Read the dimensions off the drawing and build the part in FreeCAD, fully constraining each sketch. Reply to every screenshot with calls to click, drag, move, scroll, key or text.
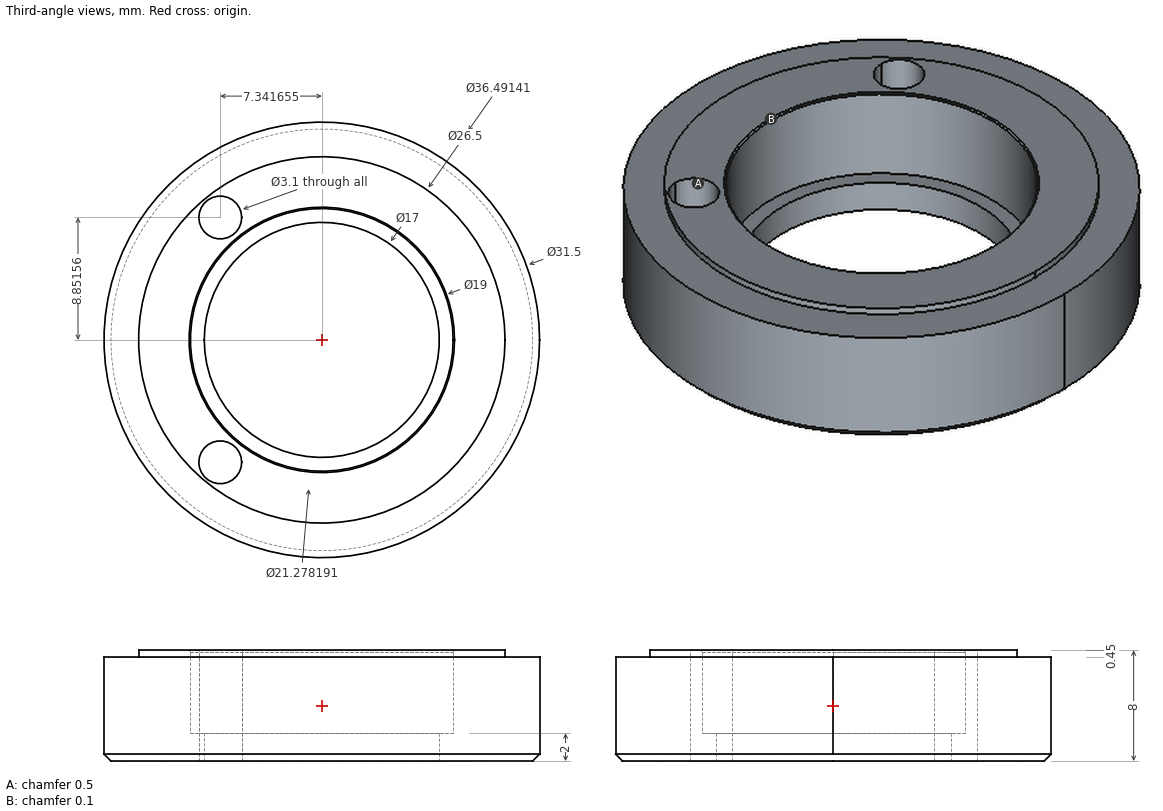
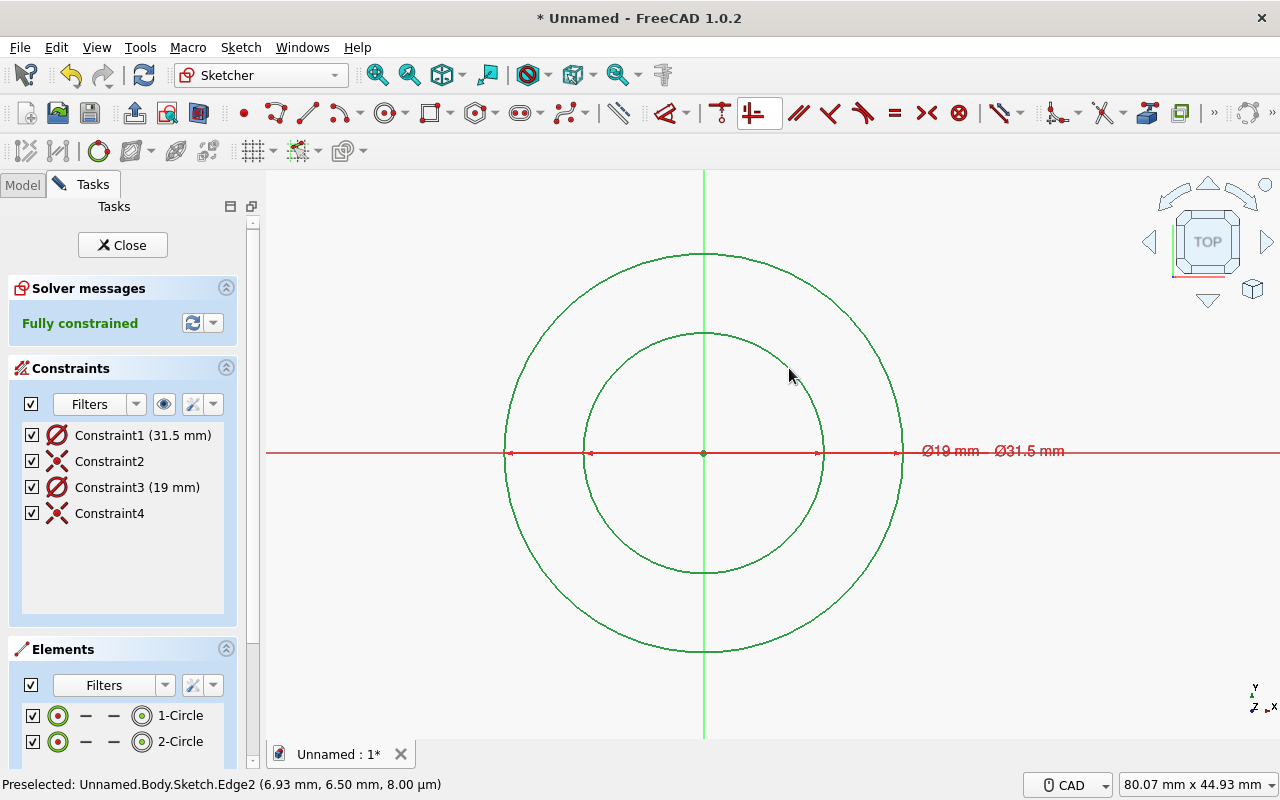
click(123, 245)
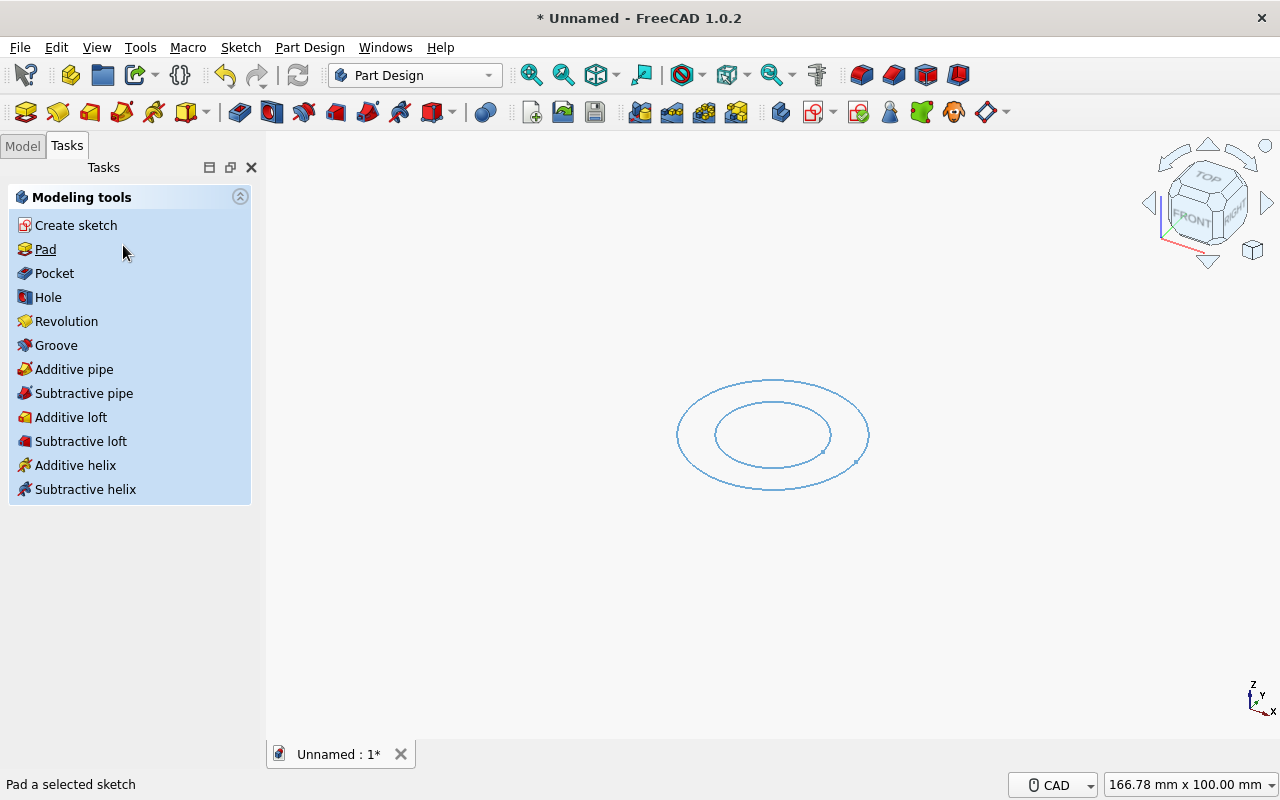
click(26, 112)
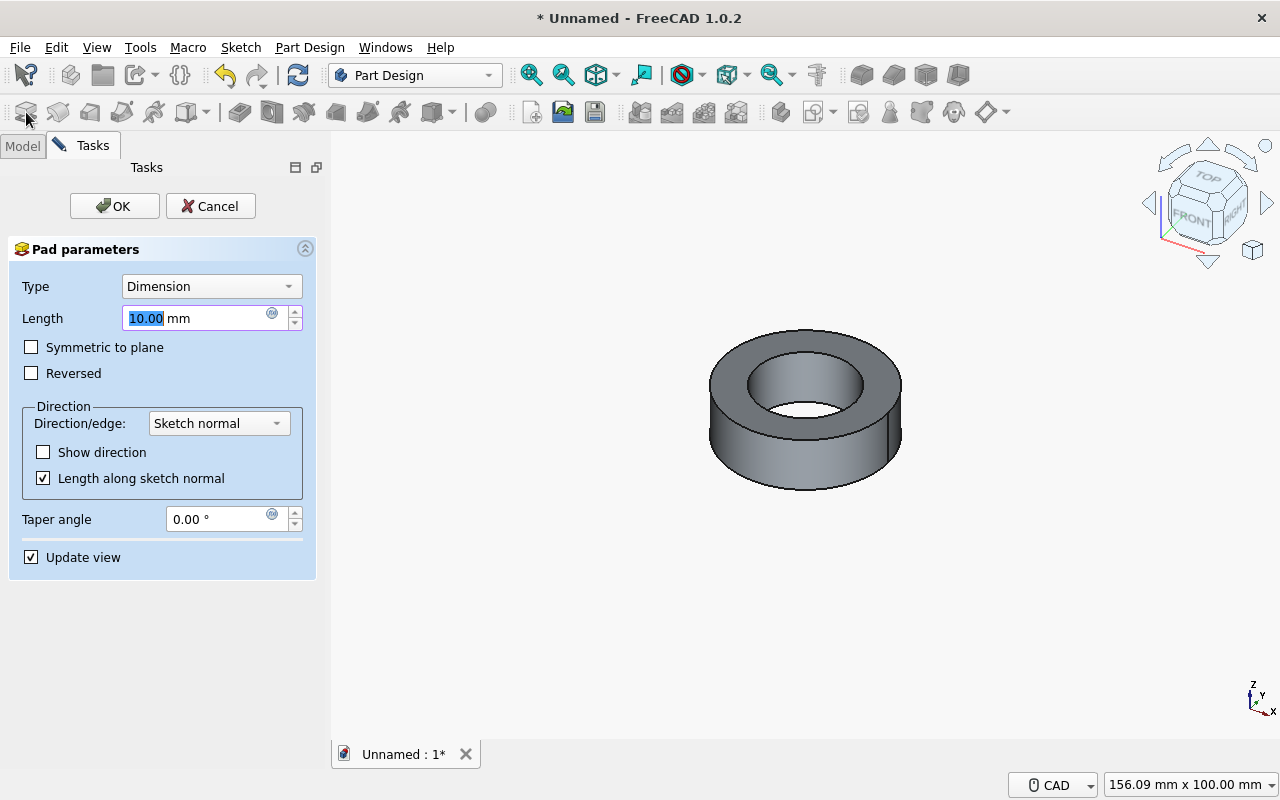
text(8)
key(Tab)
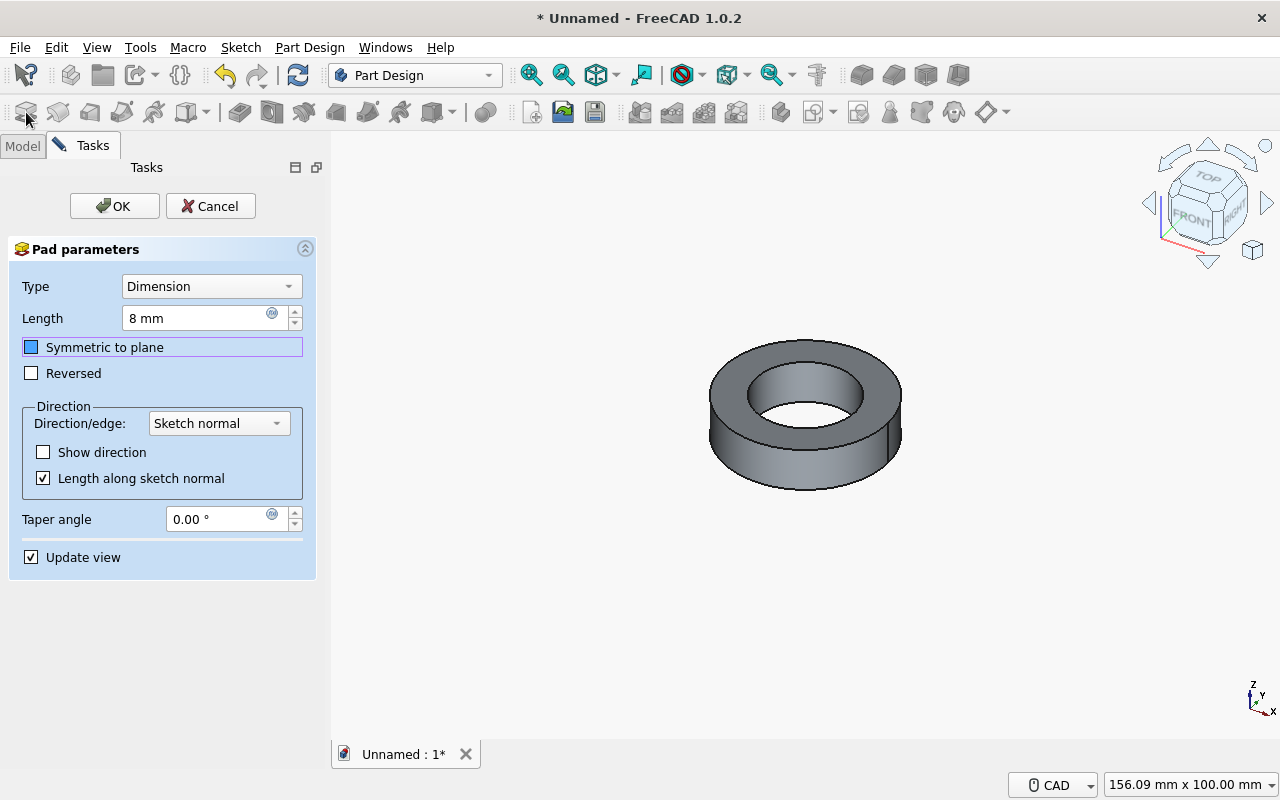
click(30, 347)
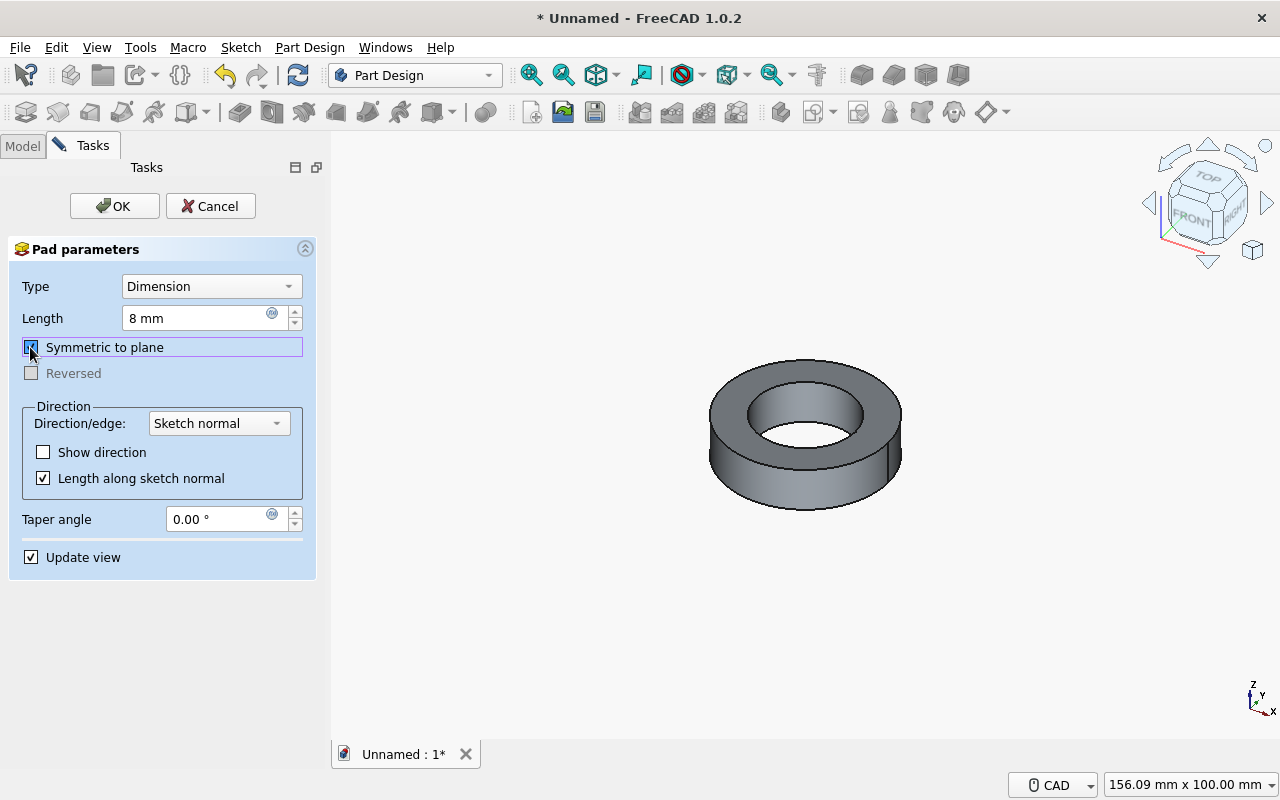
click(115, 206)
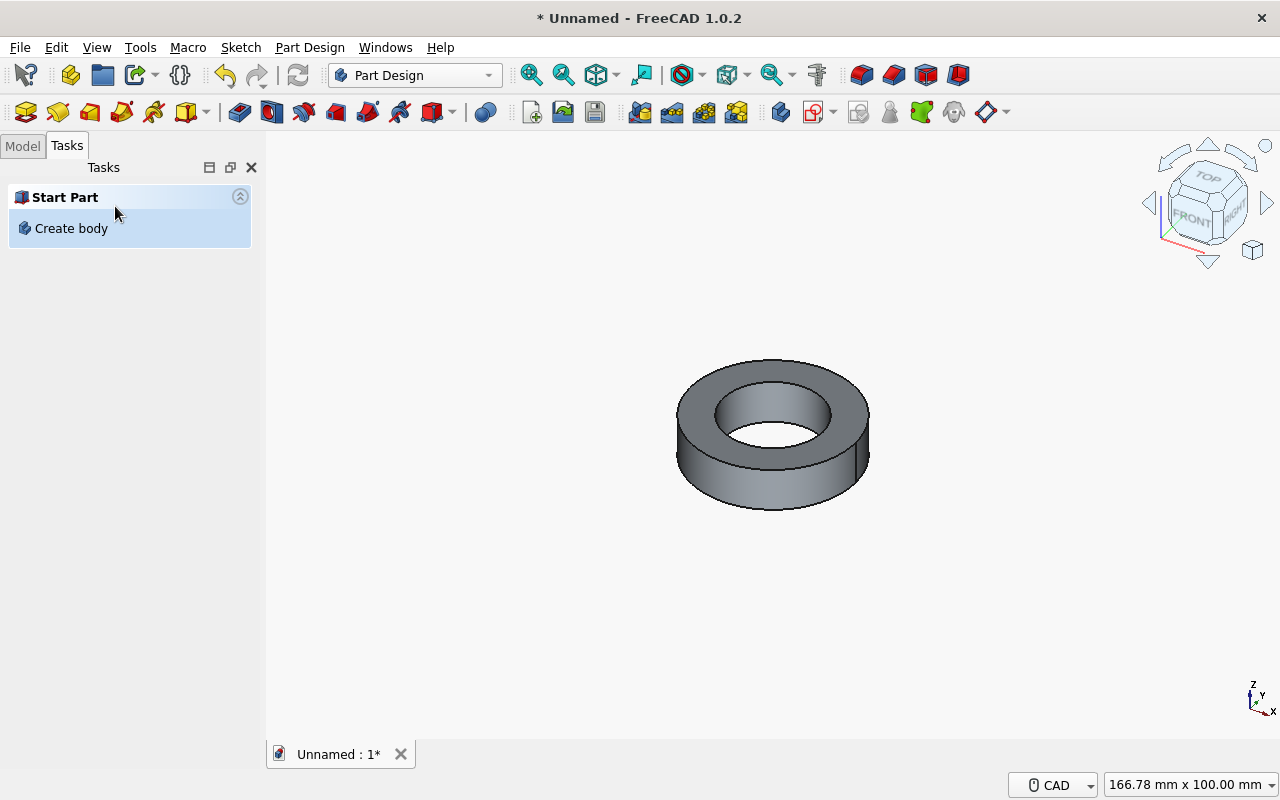
key(v)
key(f)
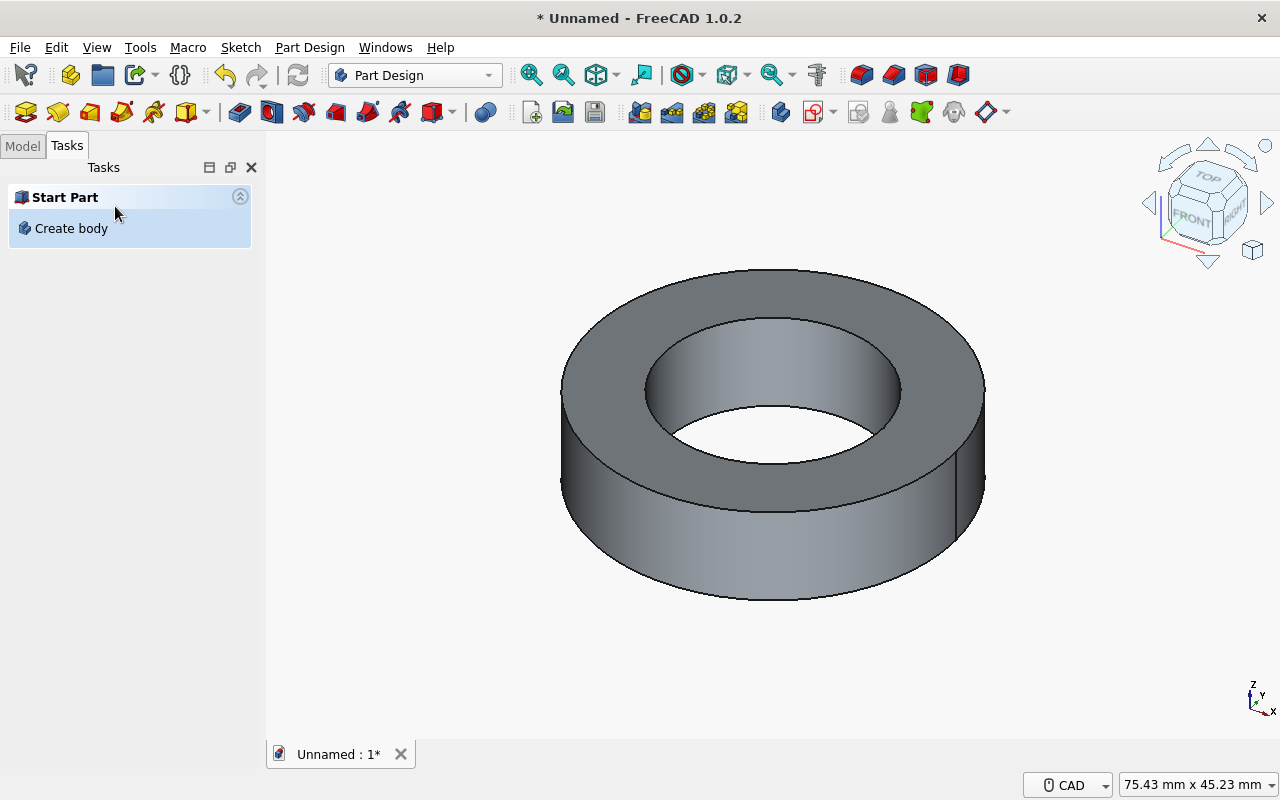
key(5)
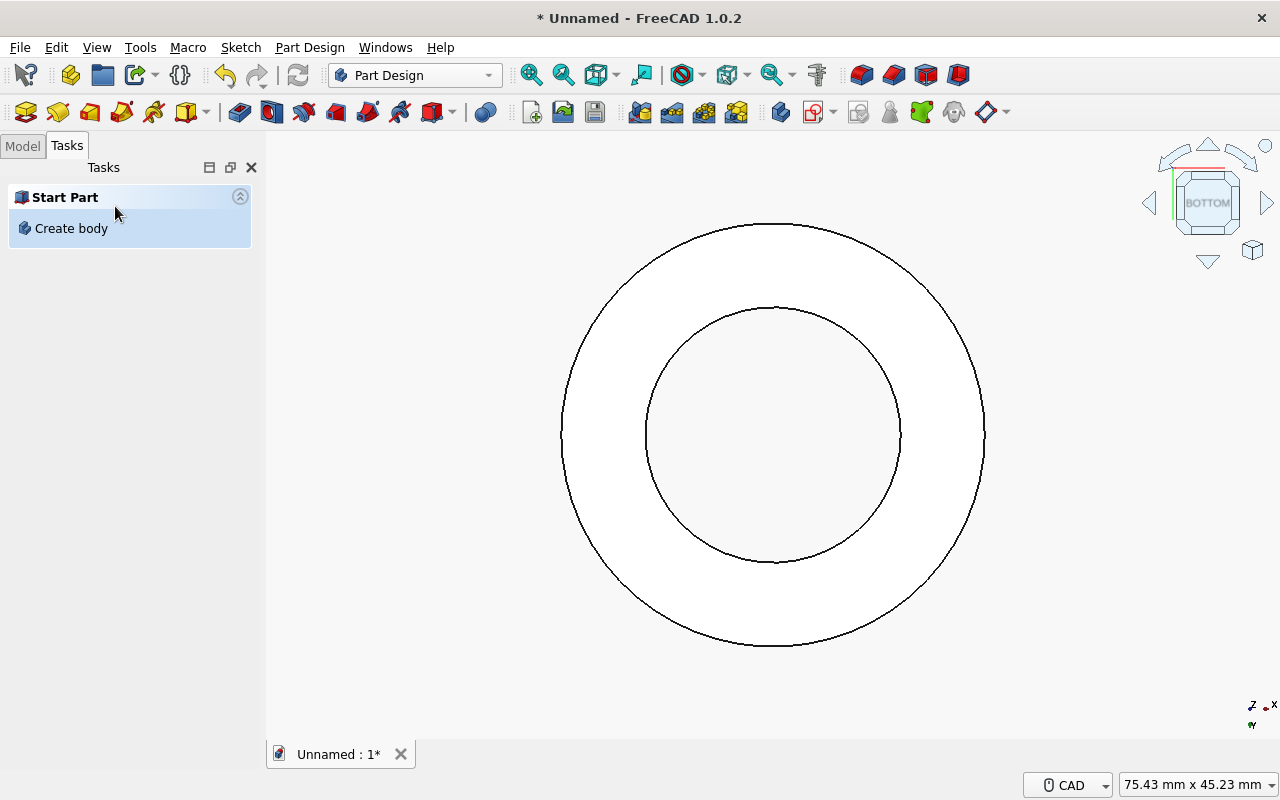
click(652, 313)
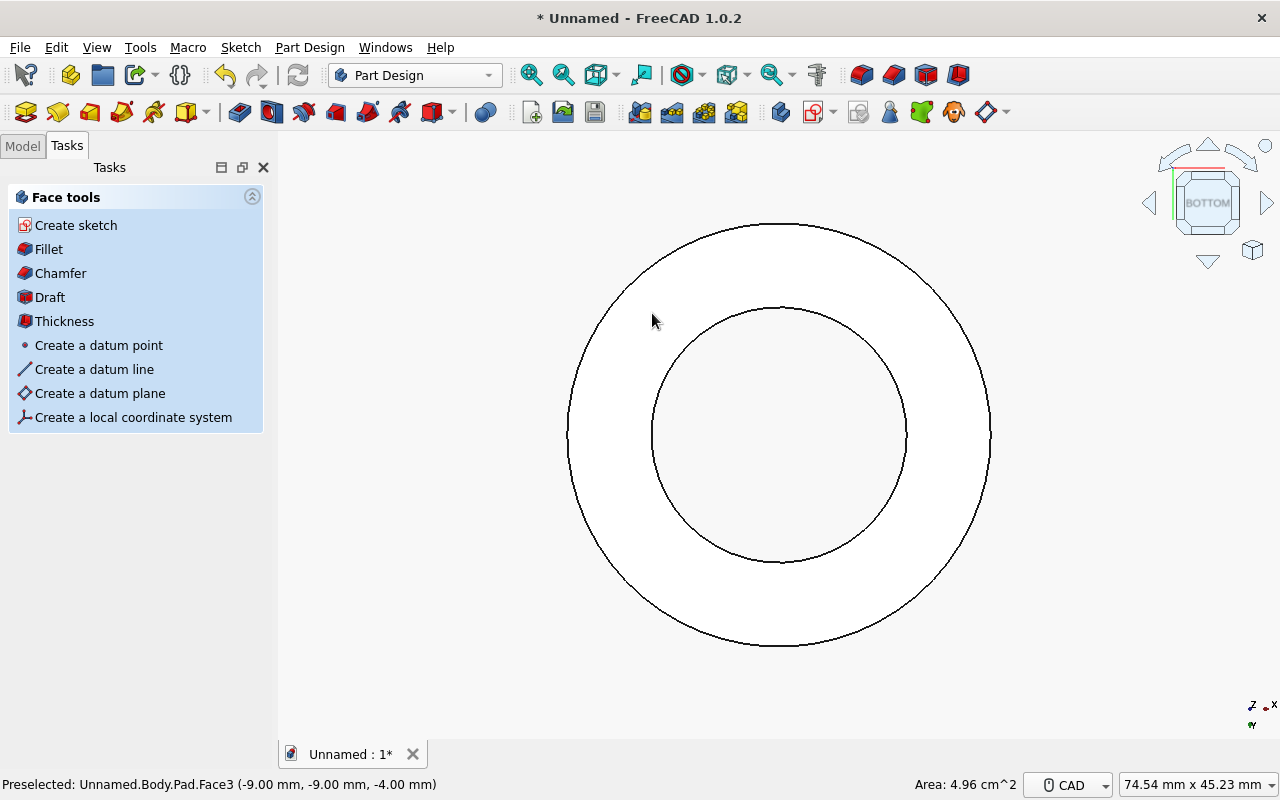
click(814, 112)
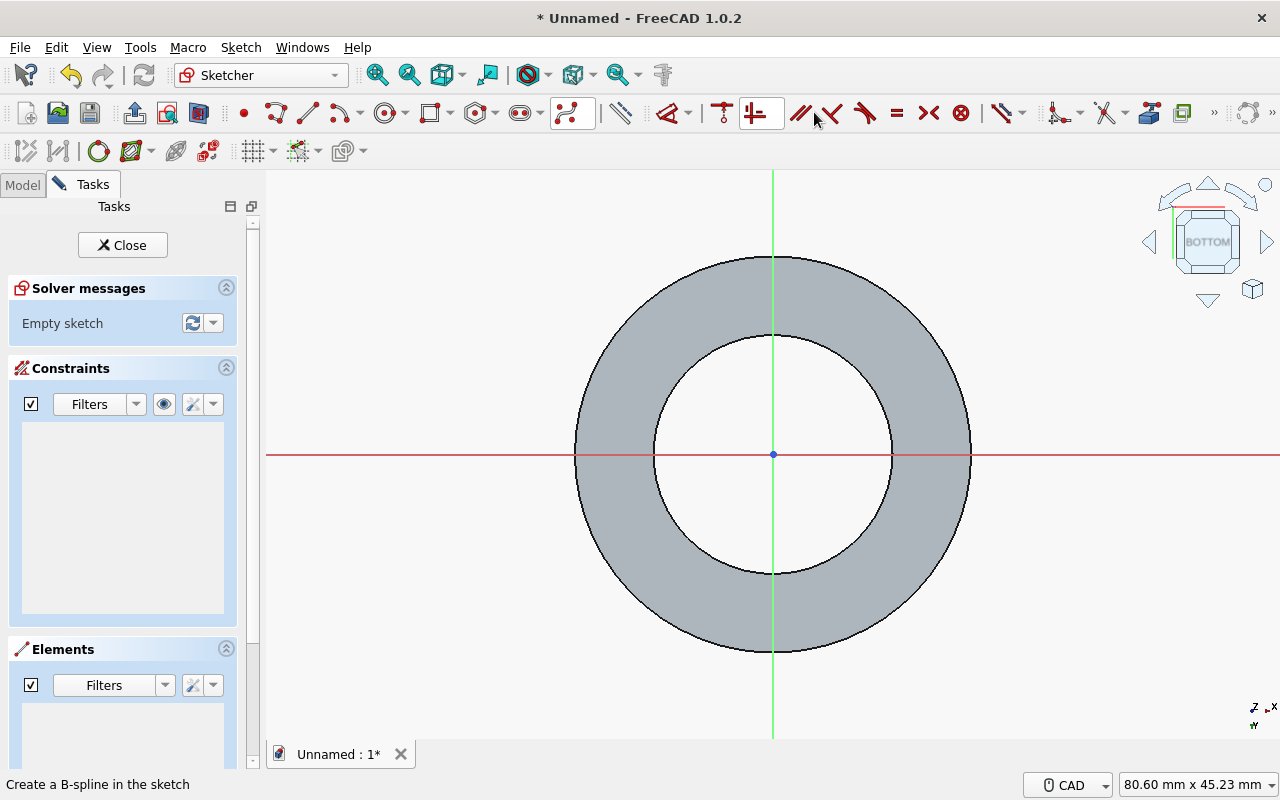
scroll(912, 455, up, 2)